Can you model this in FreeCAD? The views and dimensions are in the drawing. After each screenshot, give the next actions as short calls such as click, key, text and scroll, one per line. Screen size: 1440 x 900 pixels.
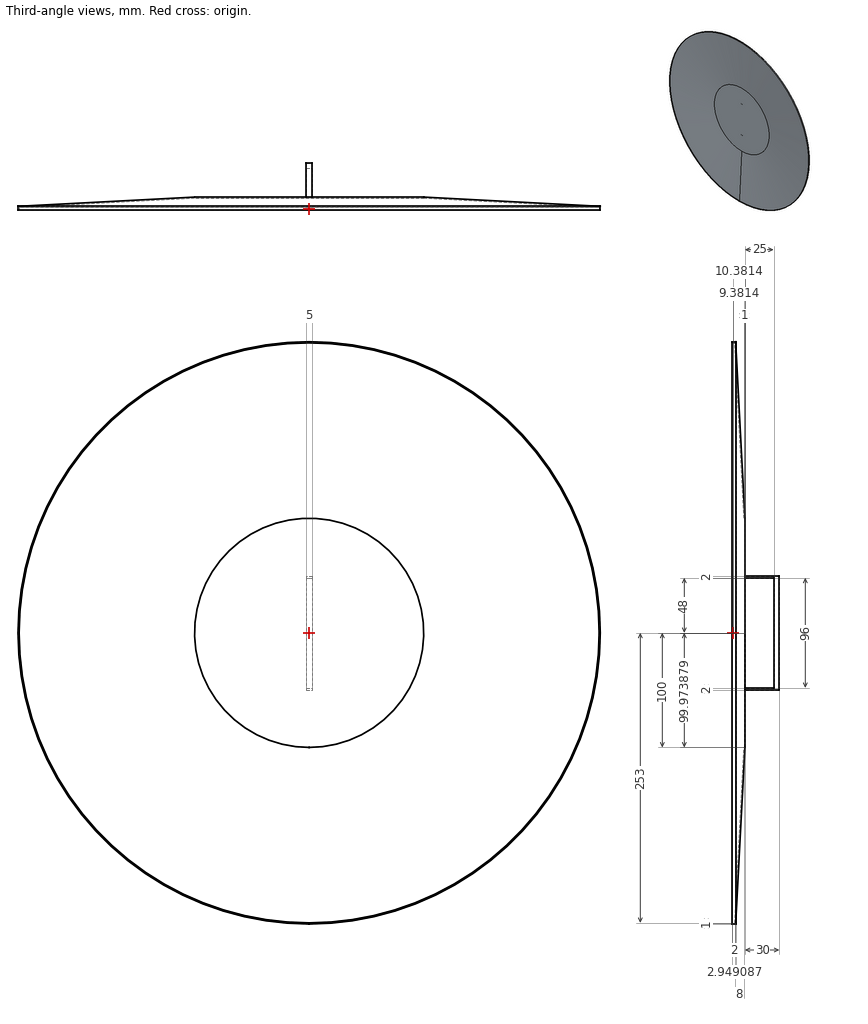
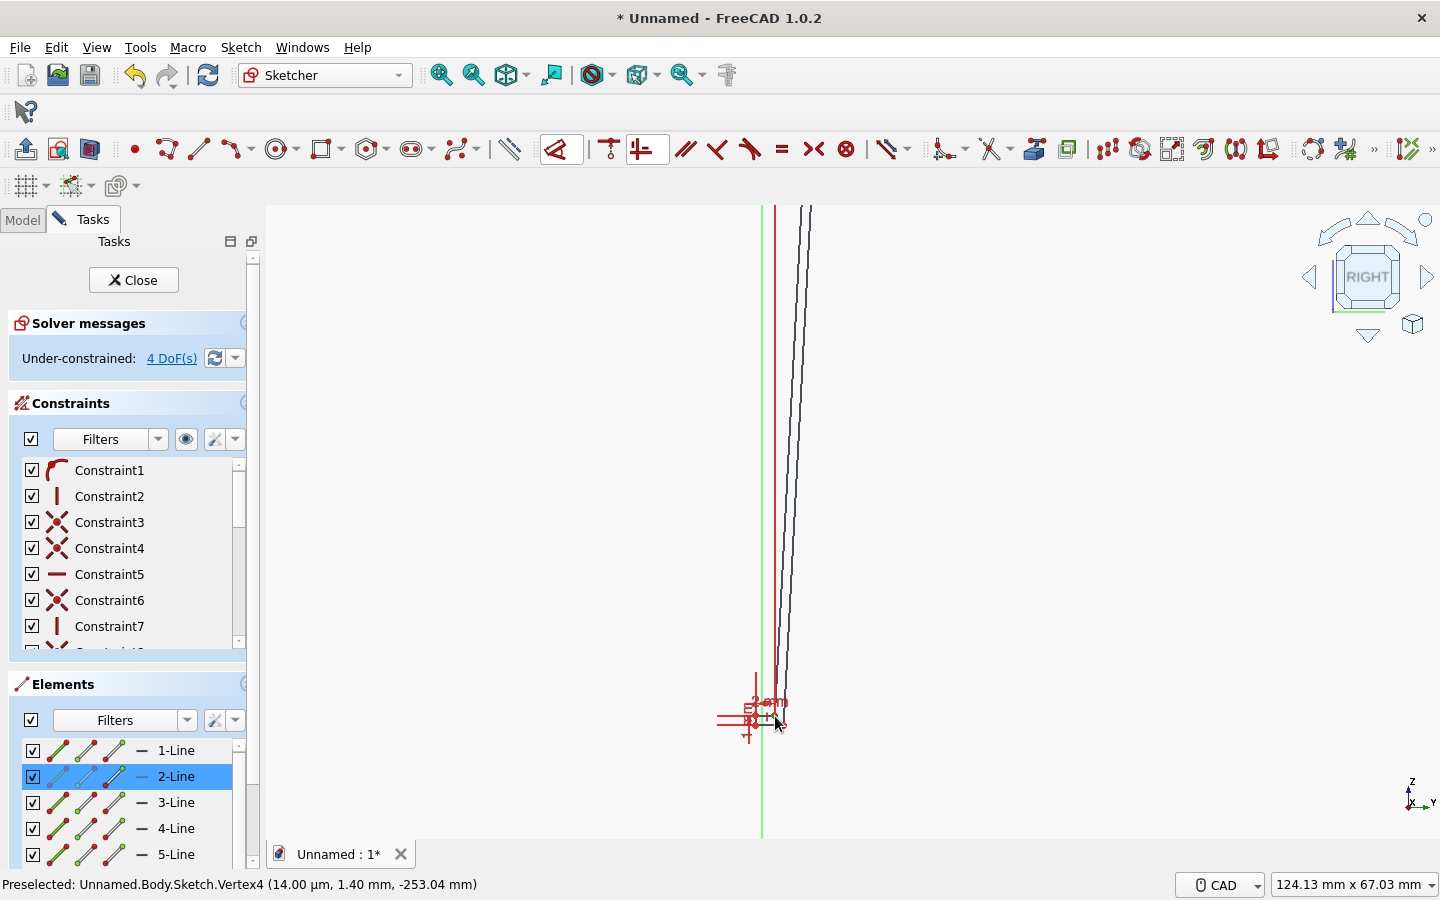
key(i)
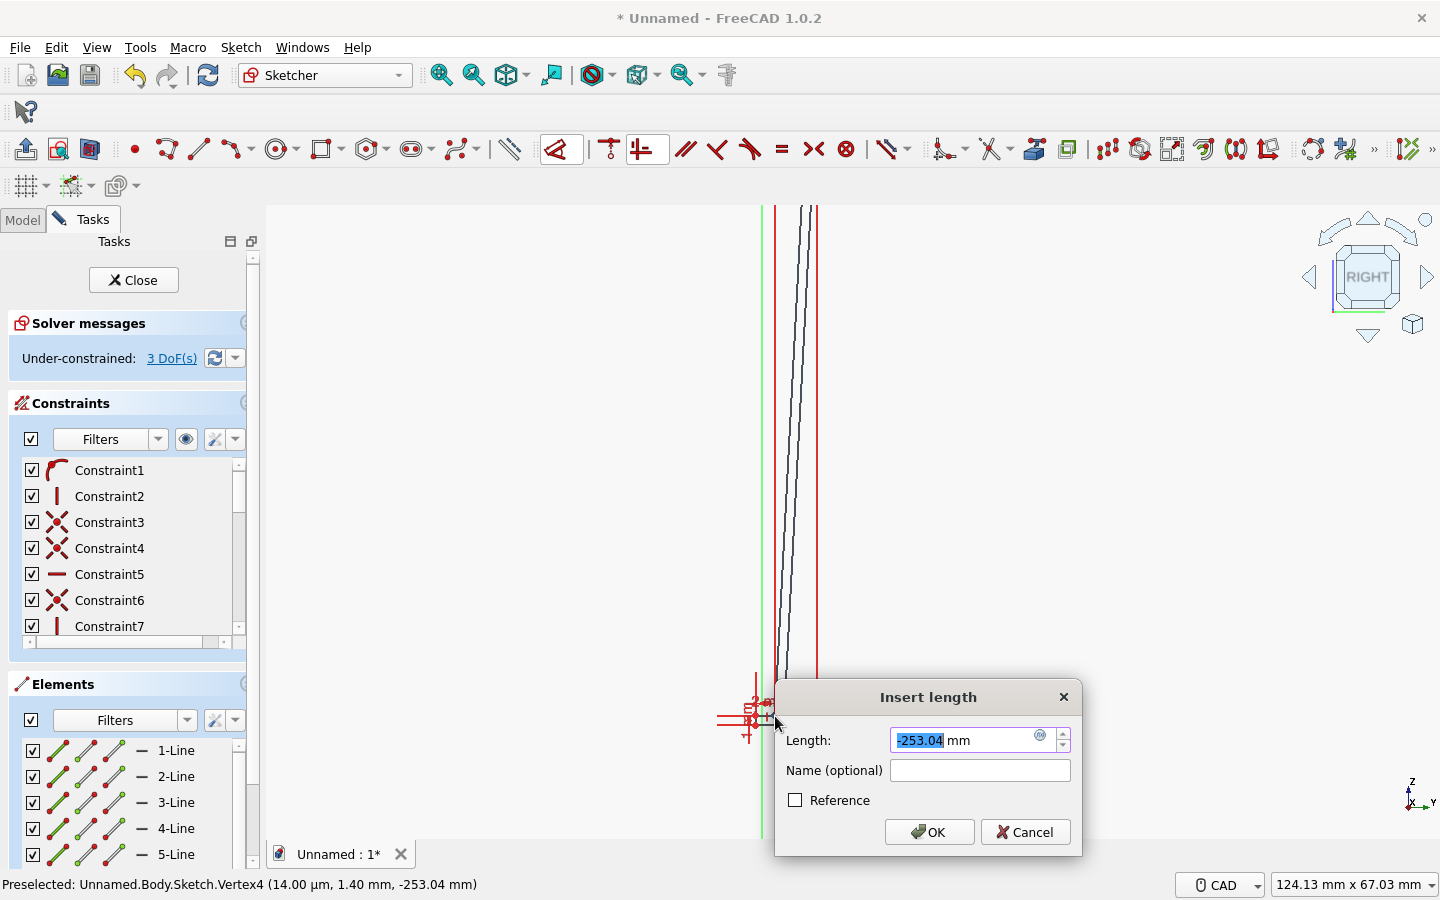
text(-253)
key(Return)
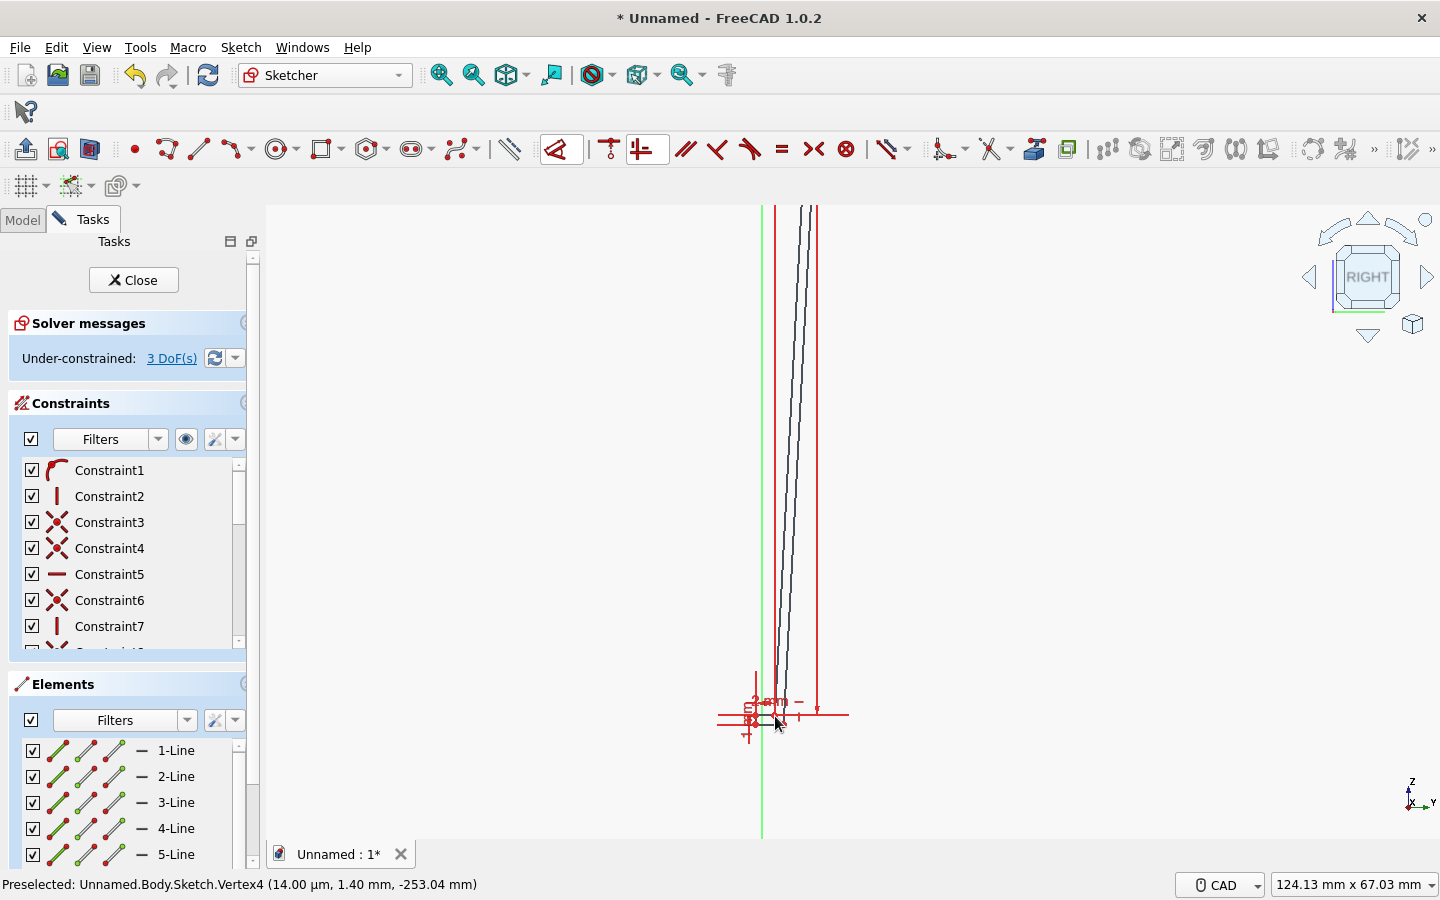
scroll(780, 720, down, 9)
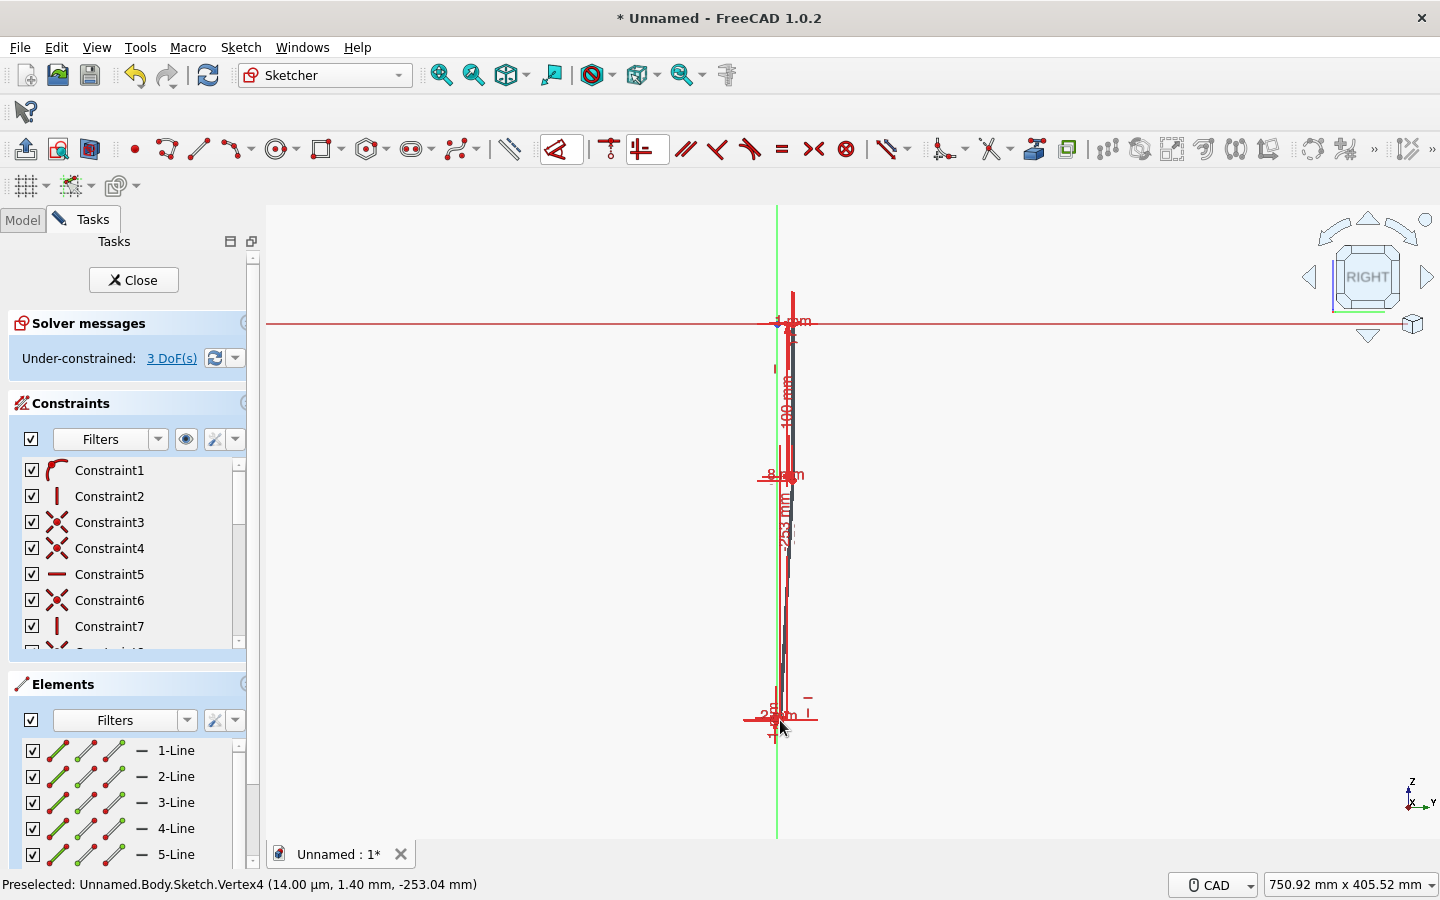
scroll(792, 324, up, 11)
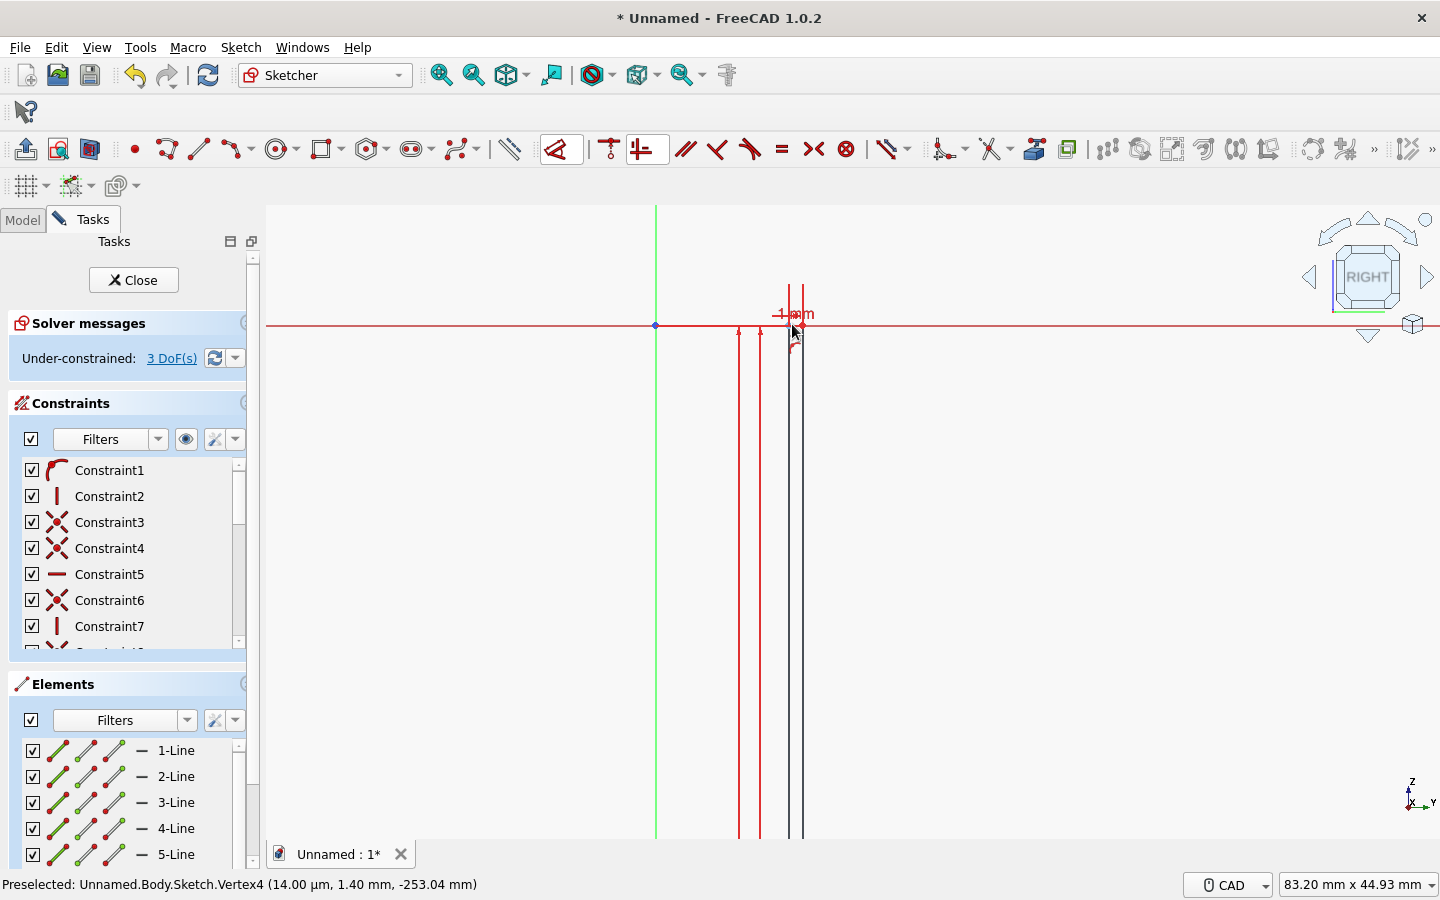
click(789, 326)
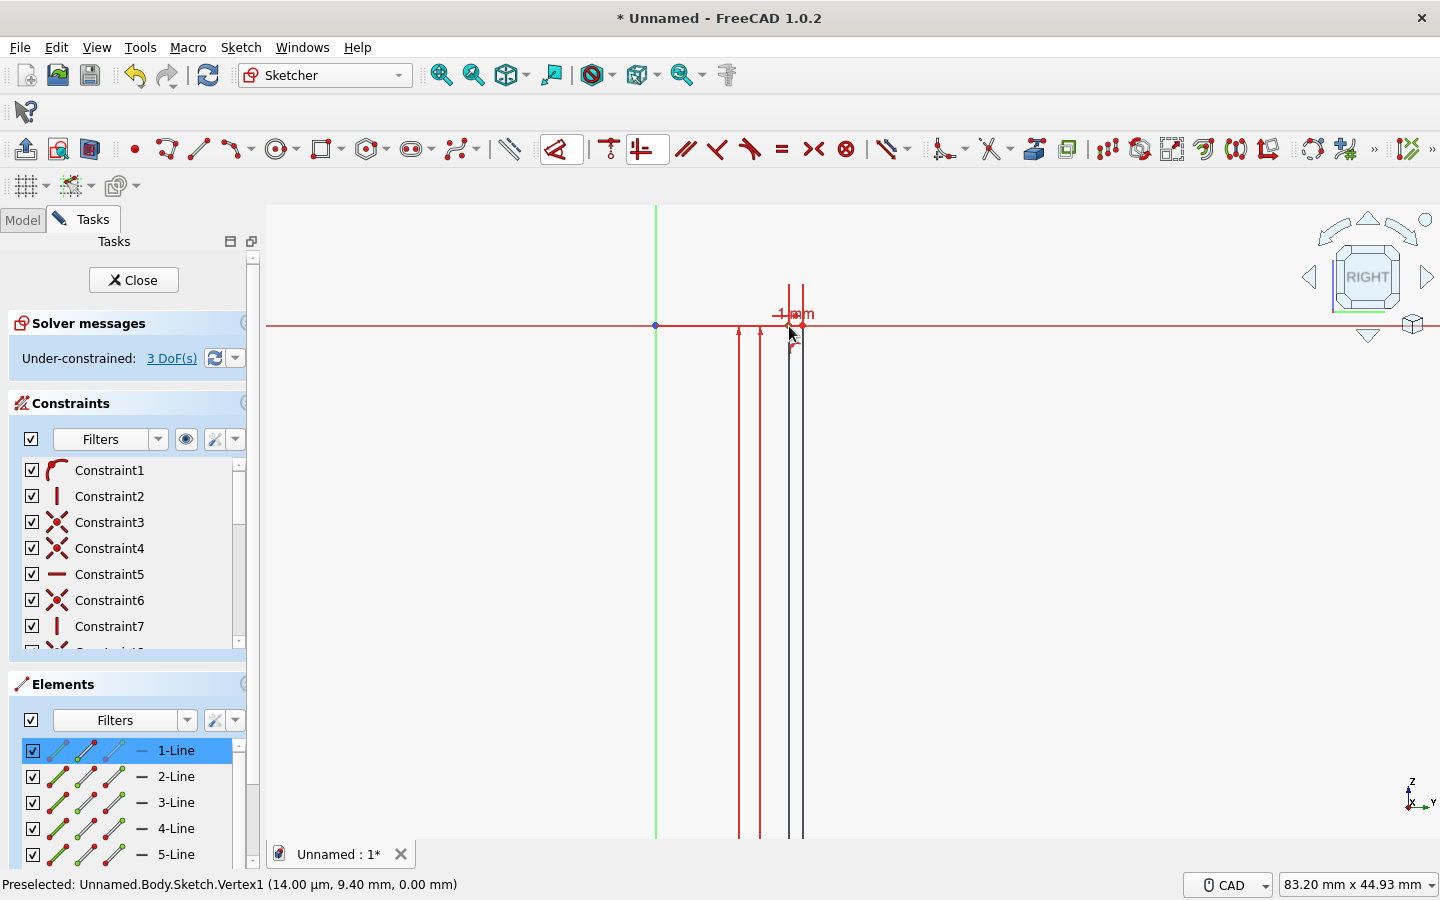
key(l)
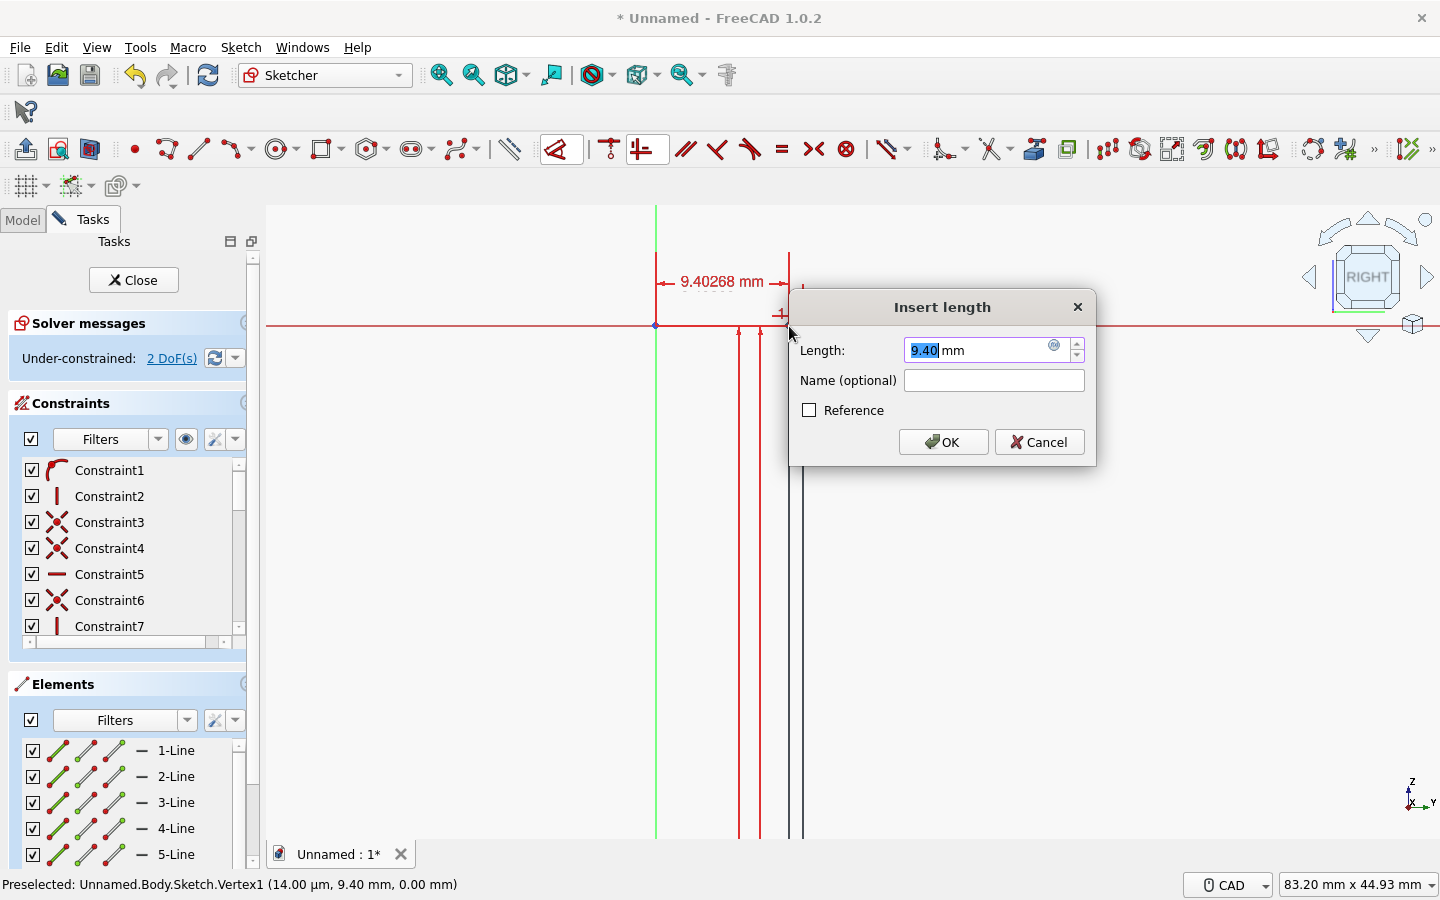
text(9.3814)
key(Return)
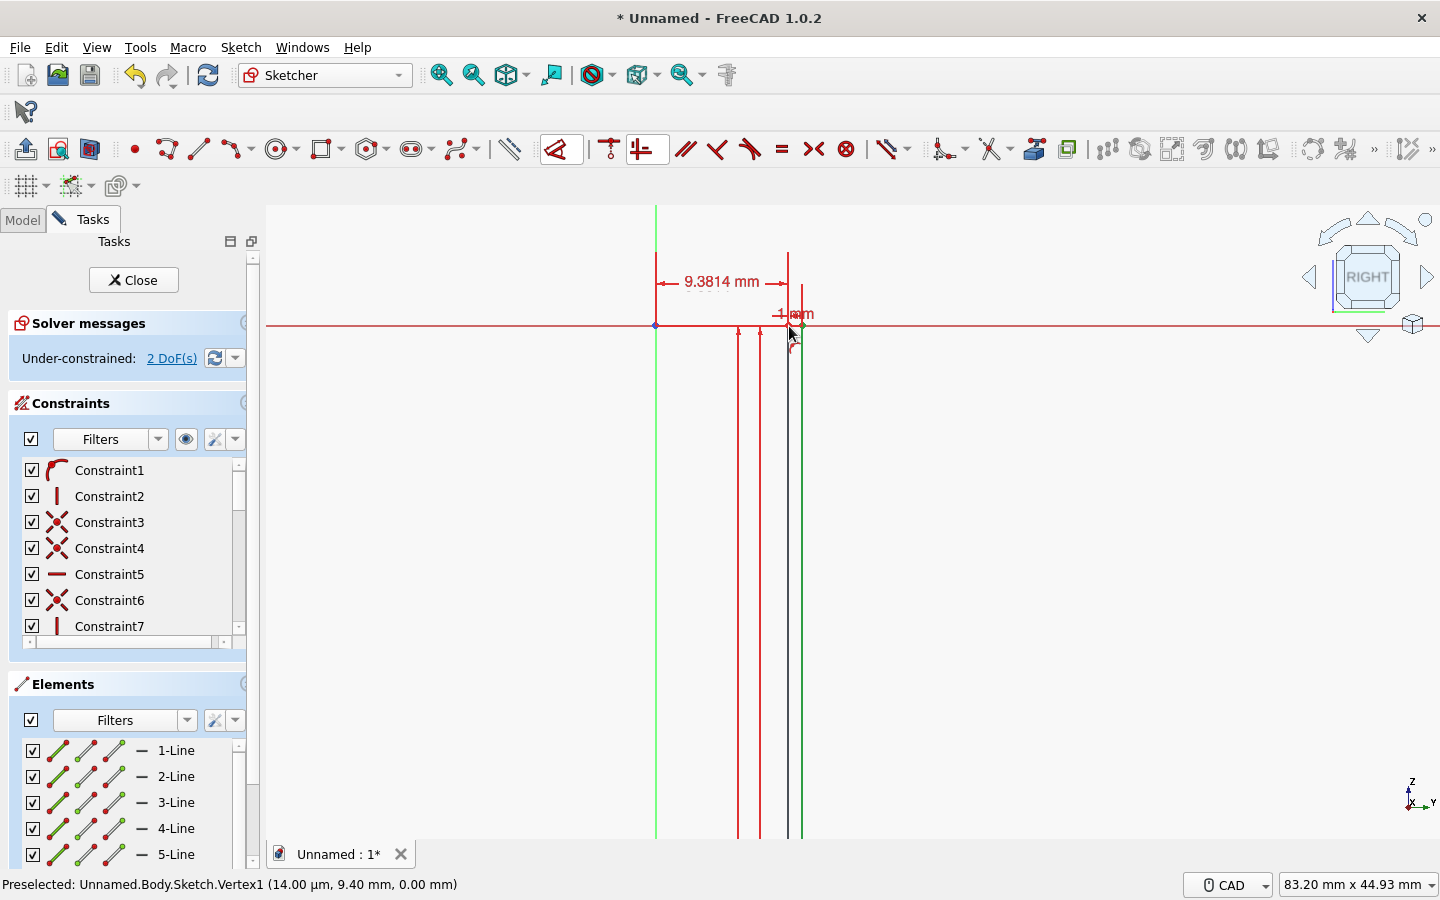
scroll(792, 323, down, 11)